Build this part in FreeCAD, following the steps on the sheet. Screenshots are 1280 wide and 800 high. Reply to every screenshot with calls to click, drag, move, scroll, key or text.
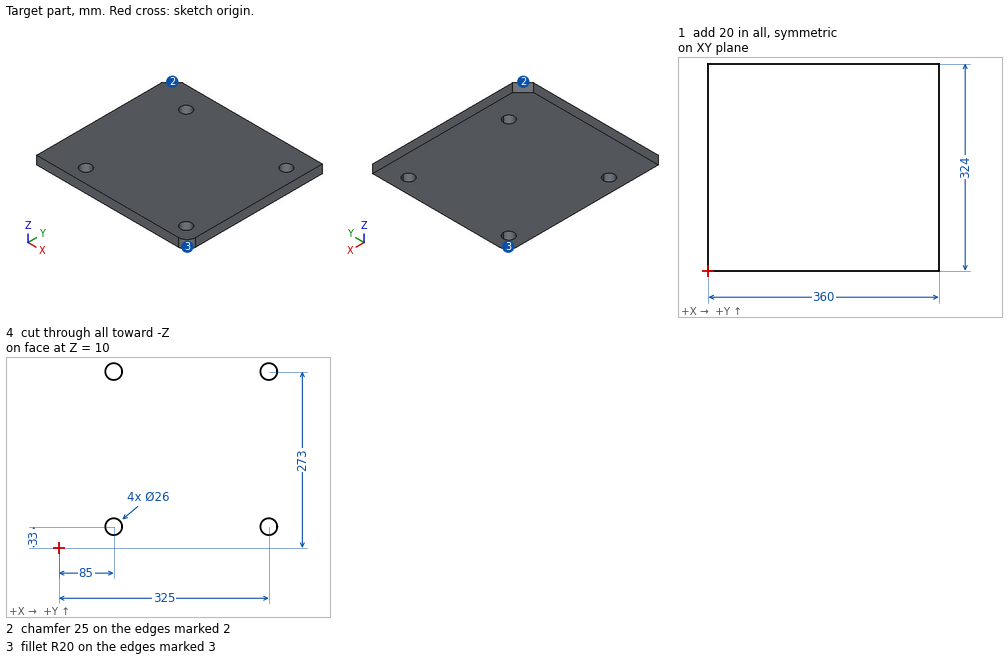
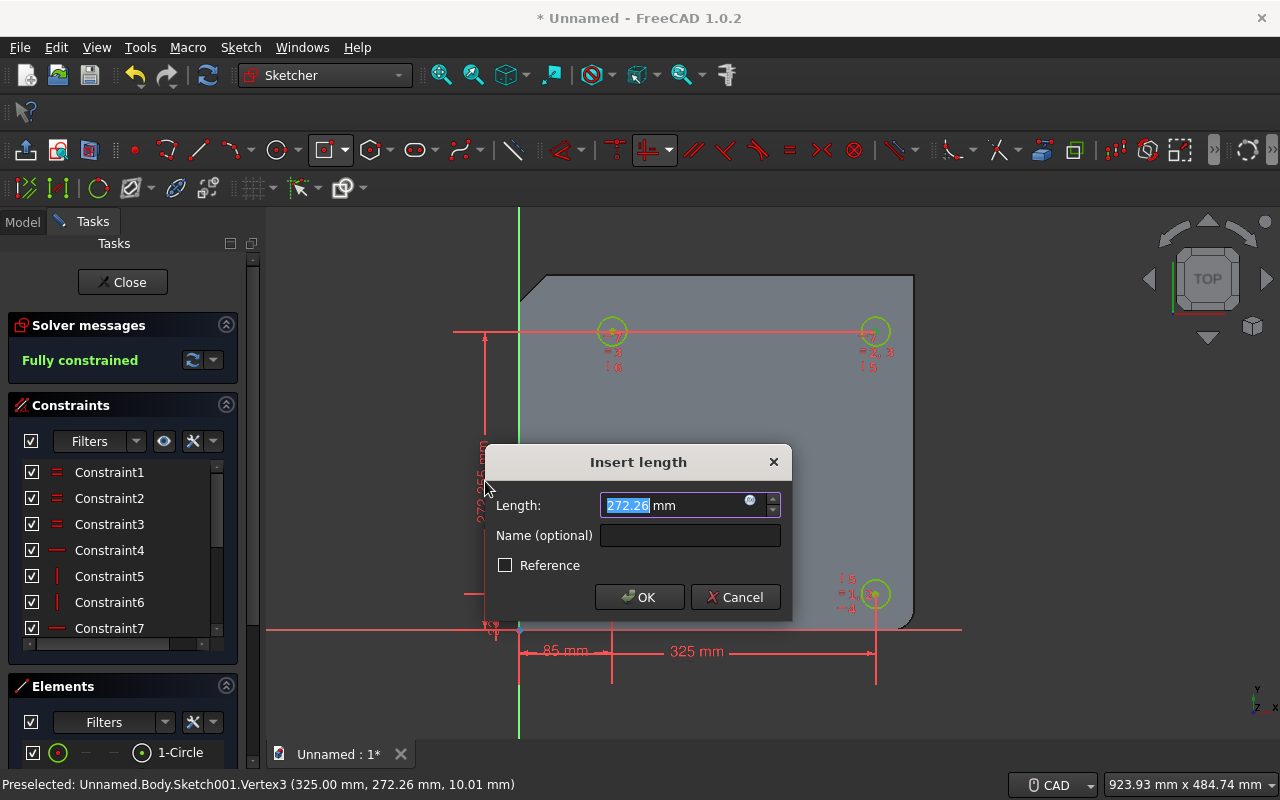
text(273)
key(Return)
key(Escape)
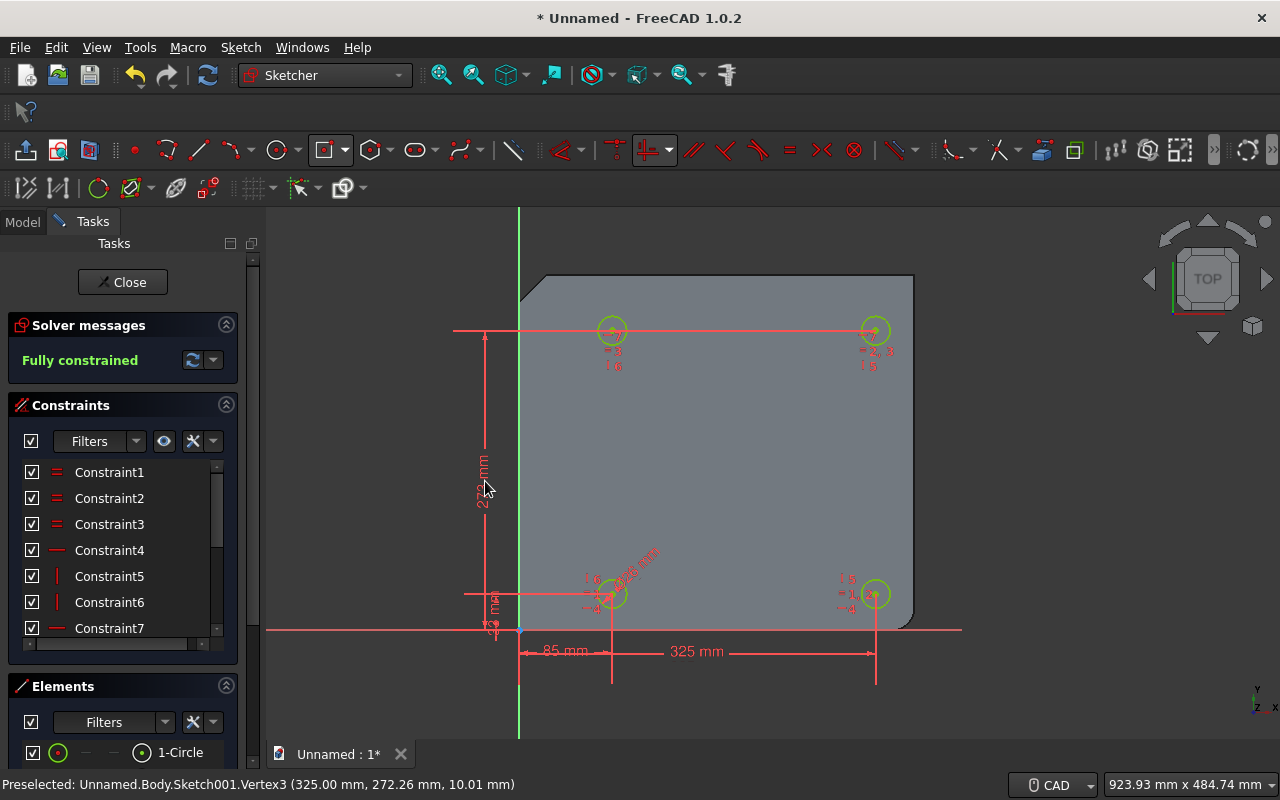
click(123, 282)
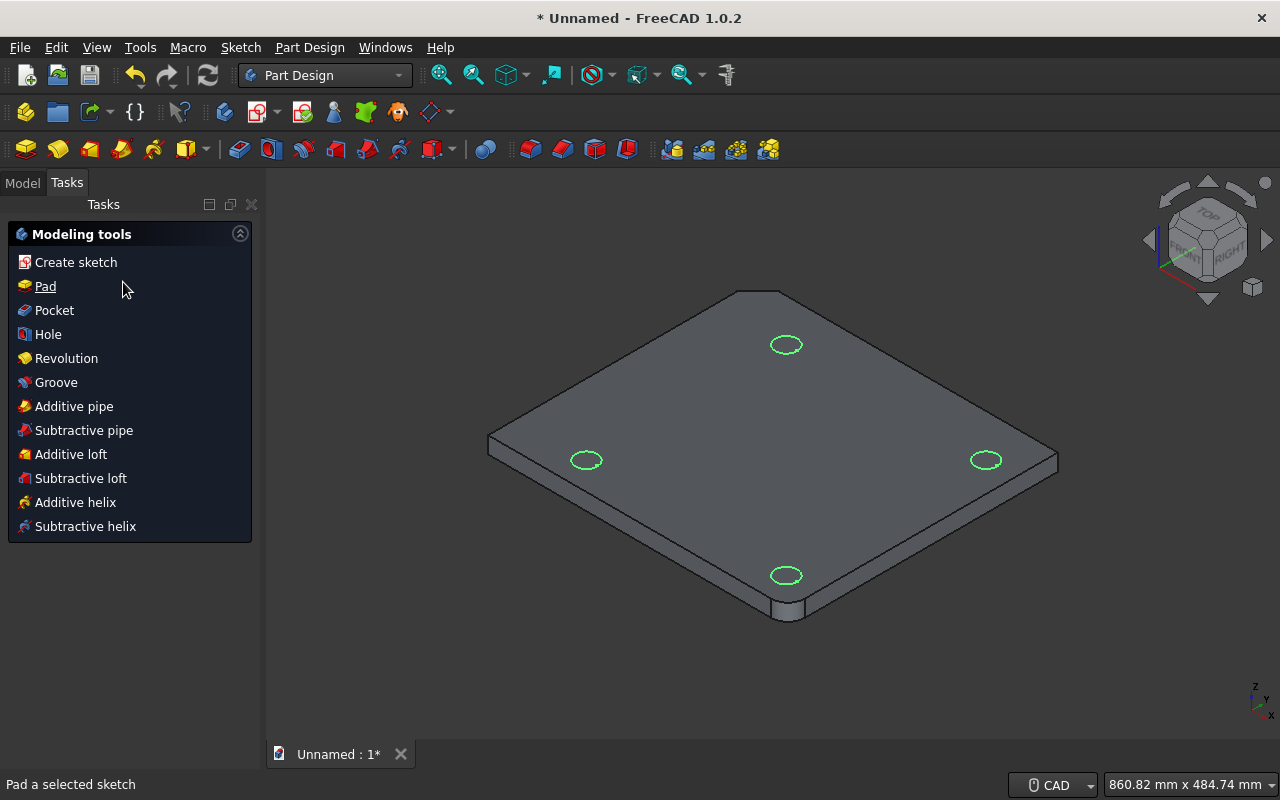
click(240, 150)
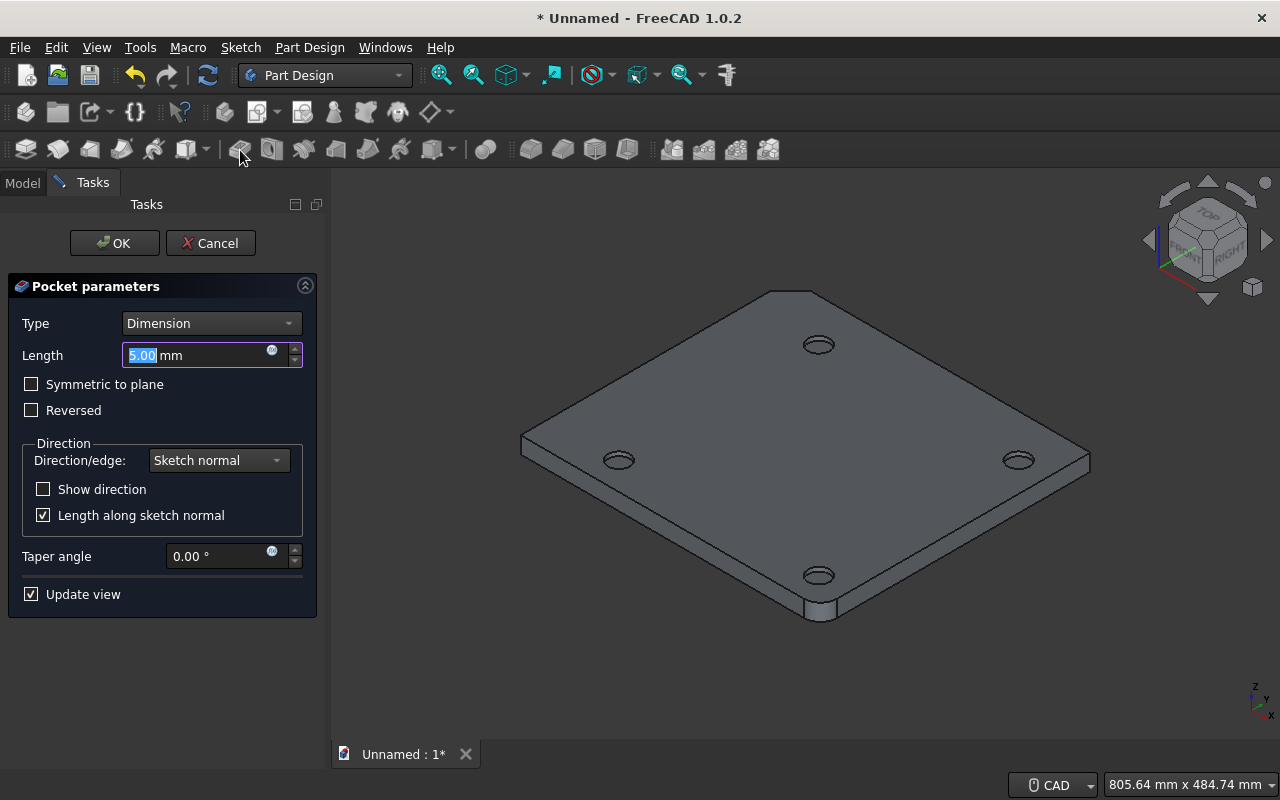
click(212, 324)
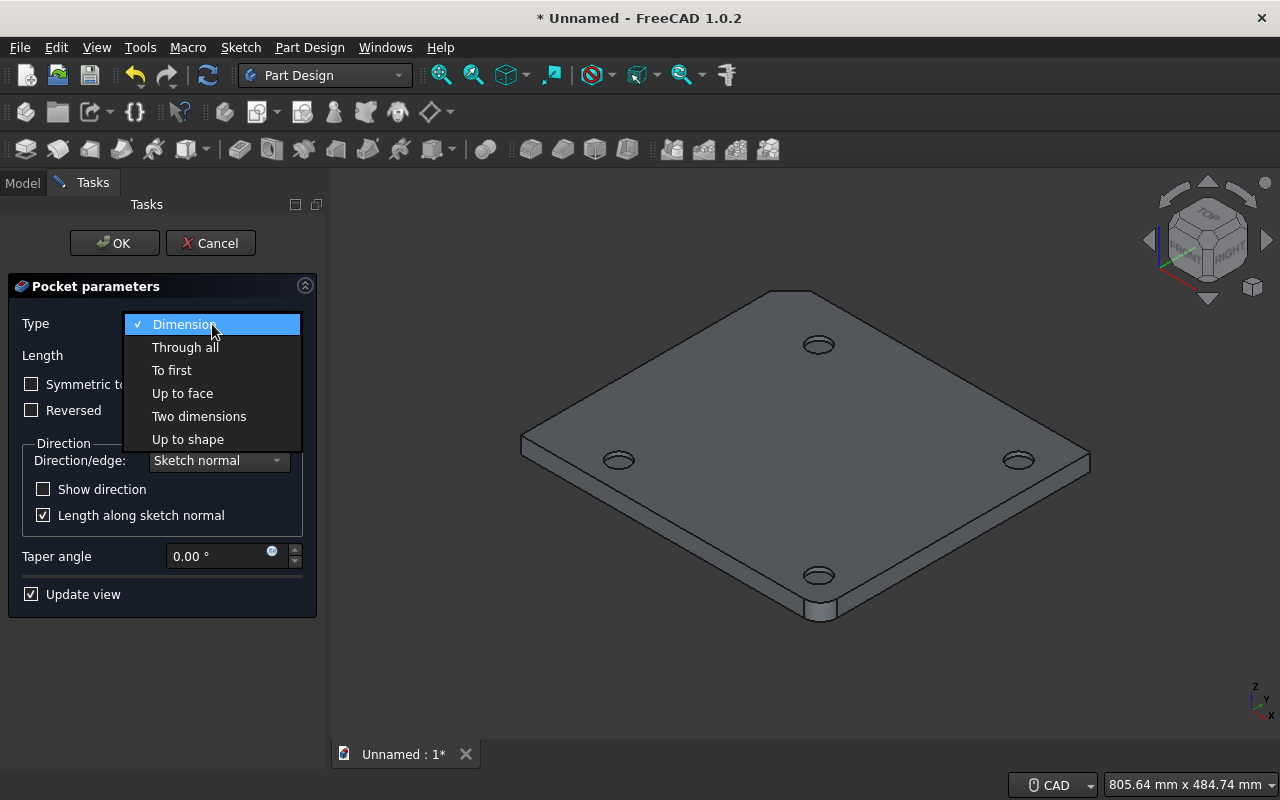
click(212, 348)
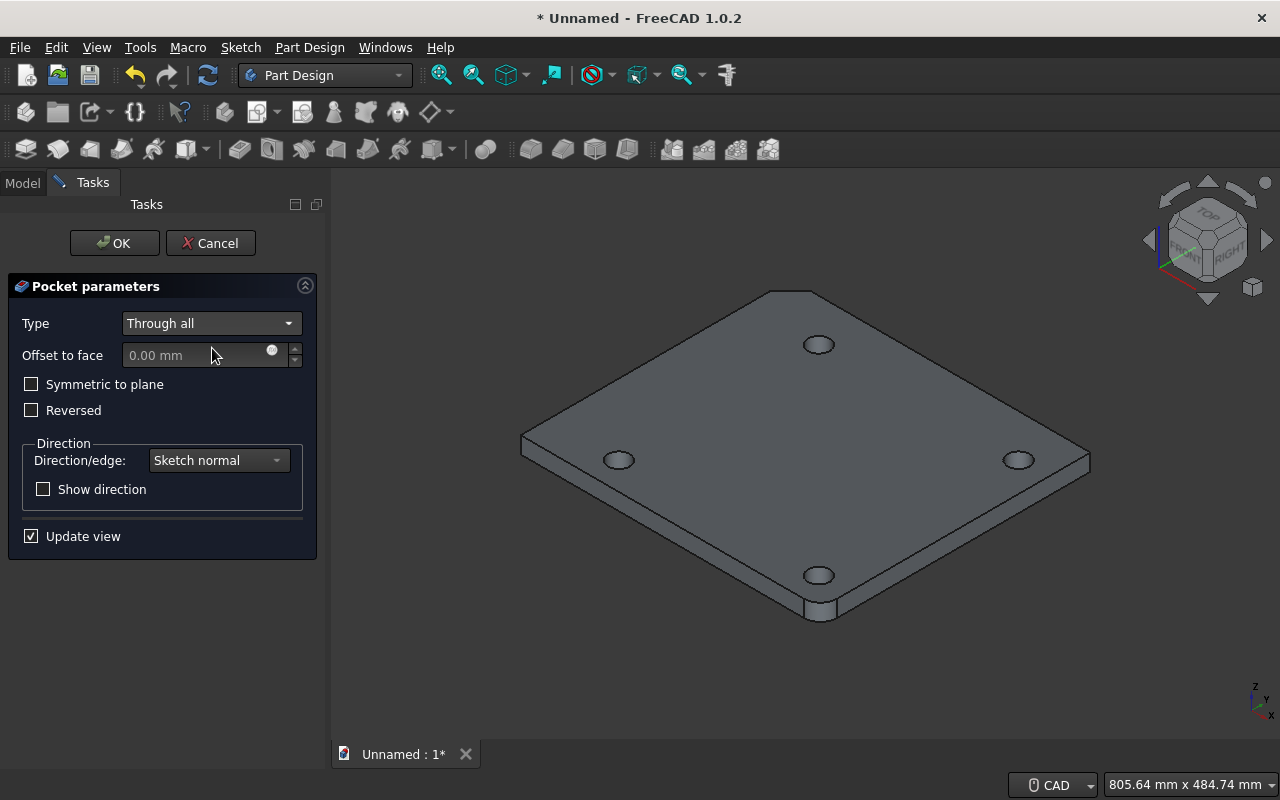
click(115, 243)